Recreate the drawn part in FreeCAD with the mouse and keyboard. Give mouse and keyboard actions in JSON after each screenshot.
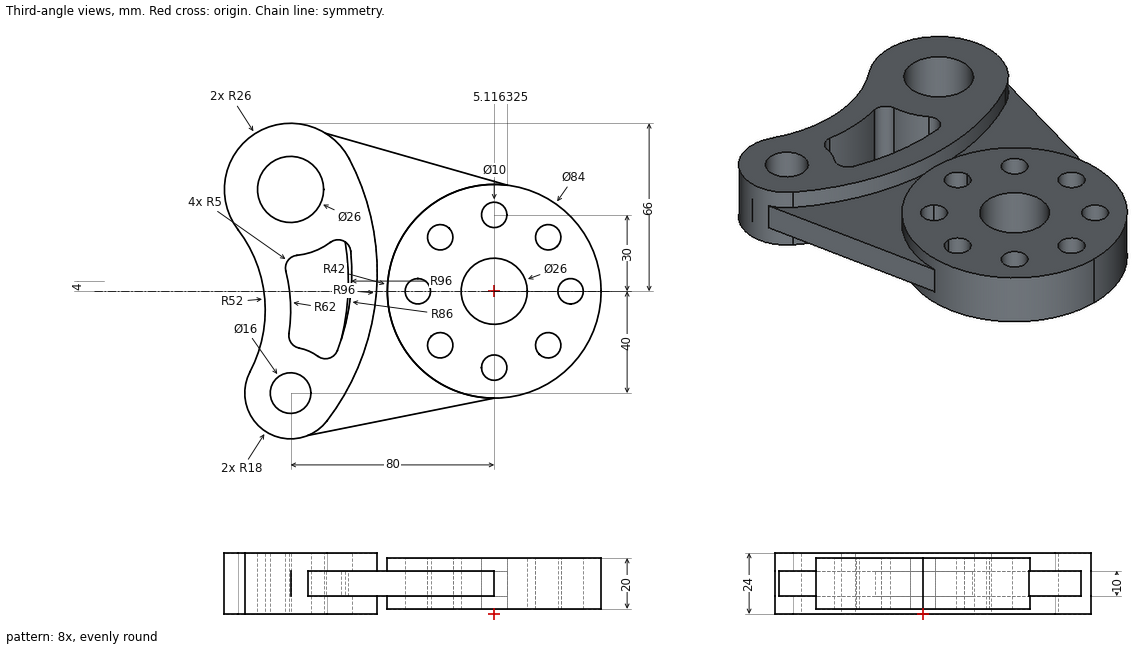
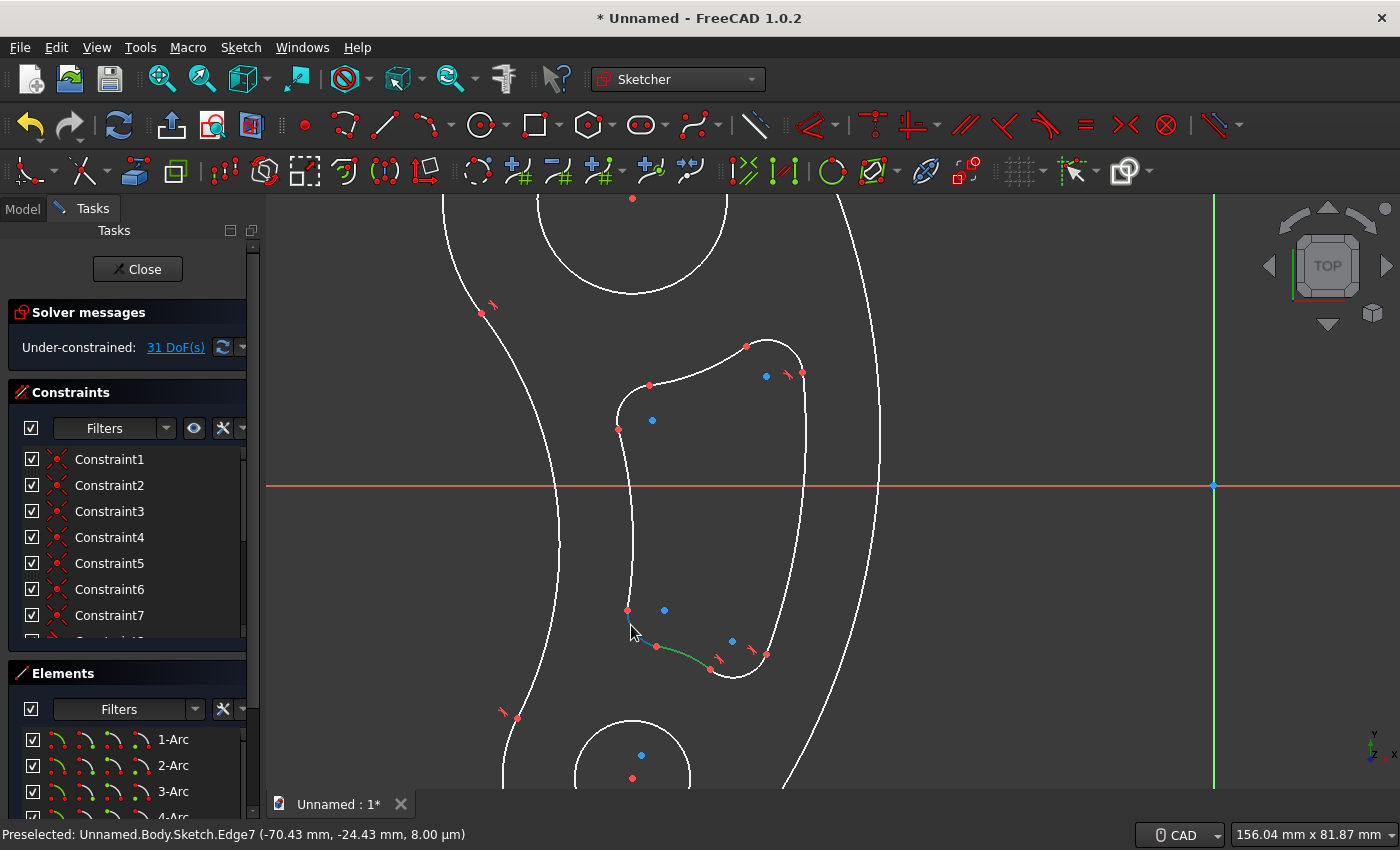
{"action": "left_click", "coordinate": [630, 625]}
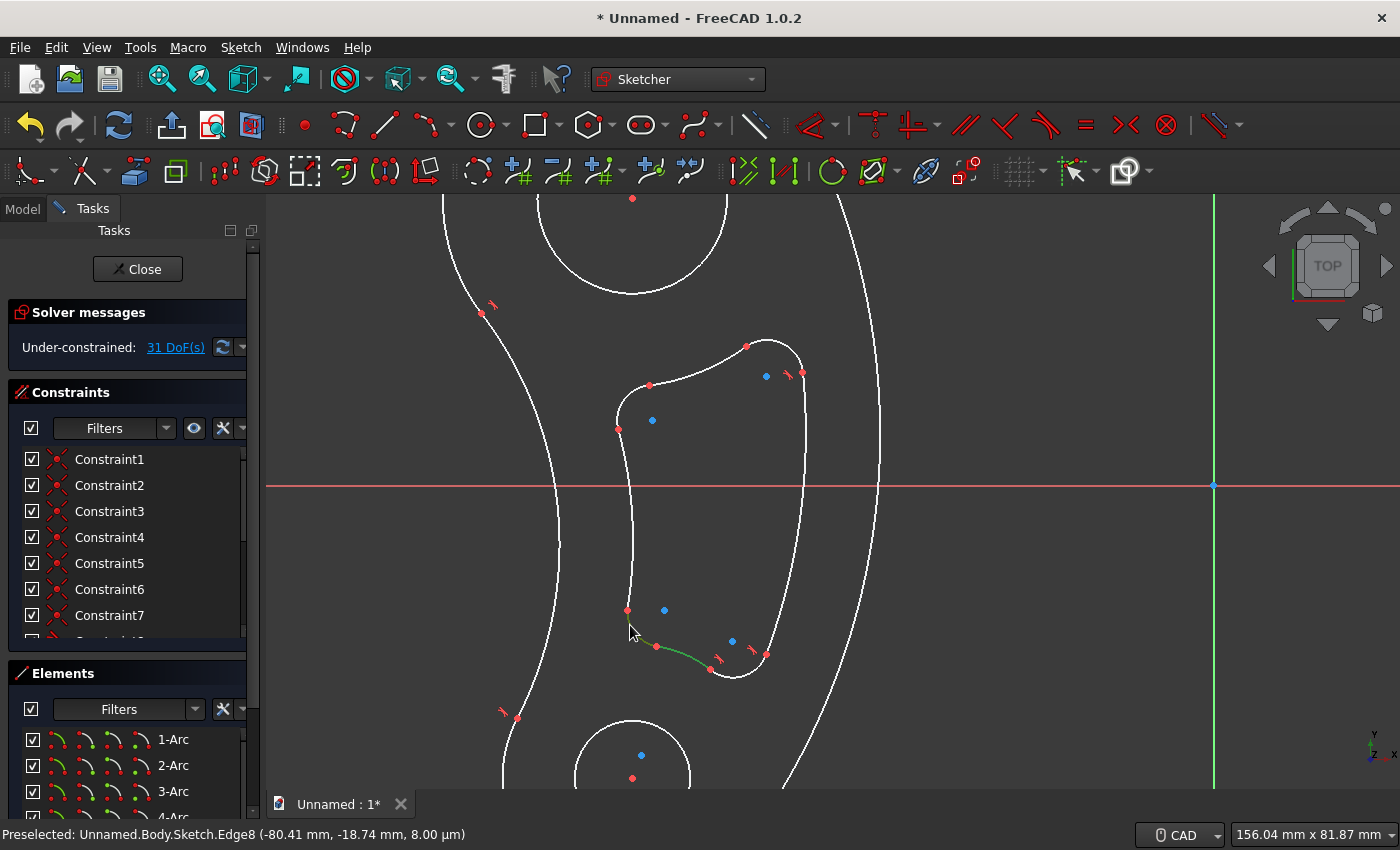
{"action": "left_click", "coordinate": [1046, 126]}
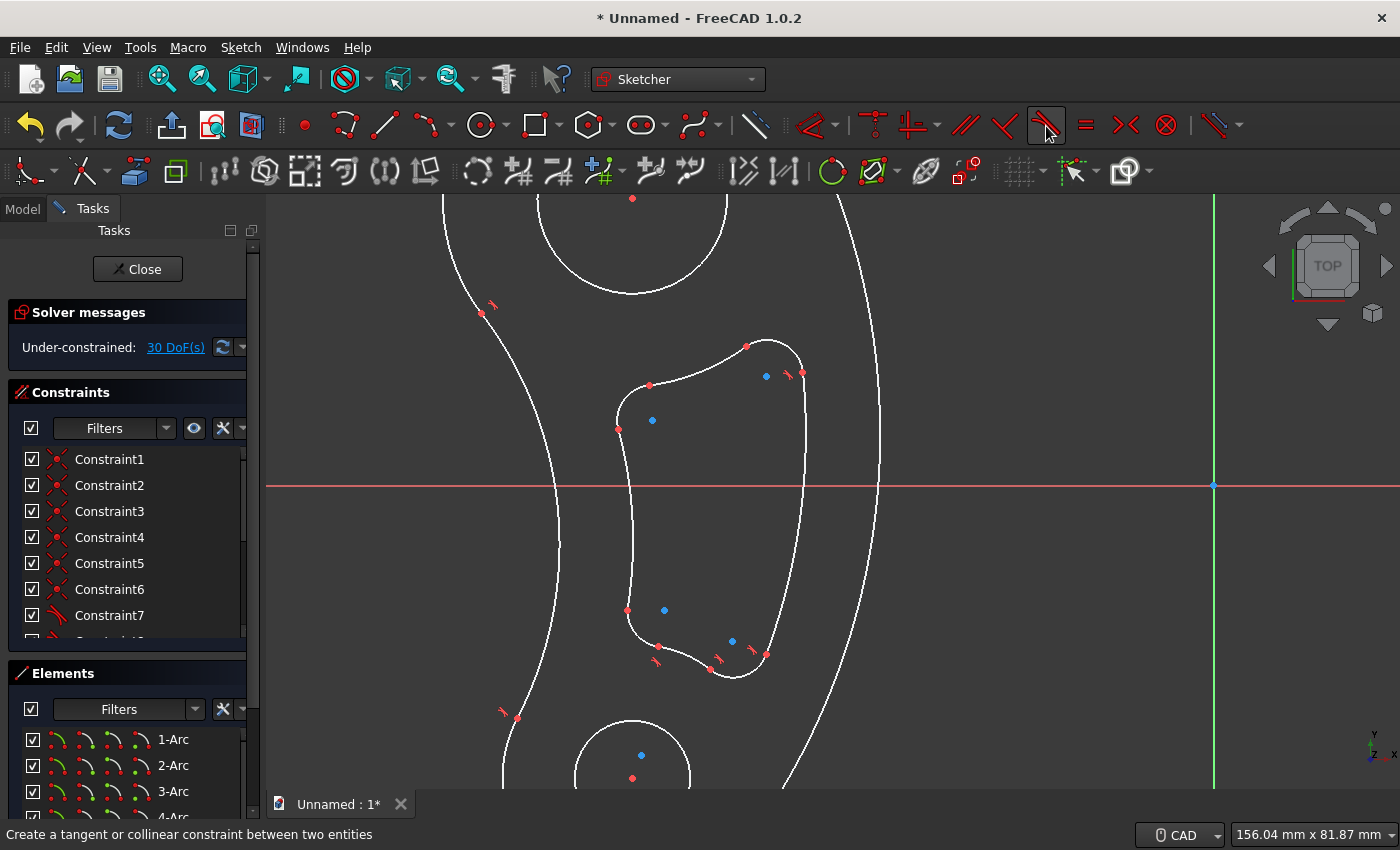
{"action": "left_click", "coordinate": [631, 625]}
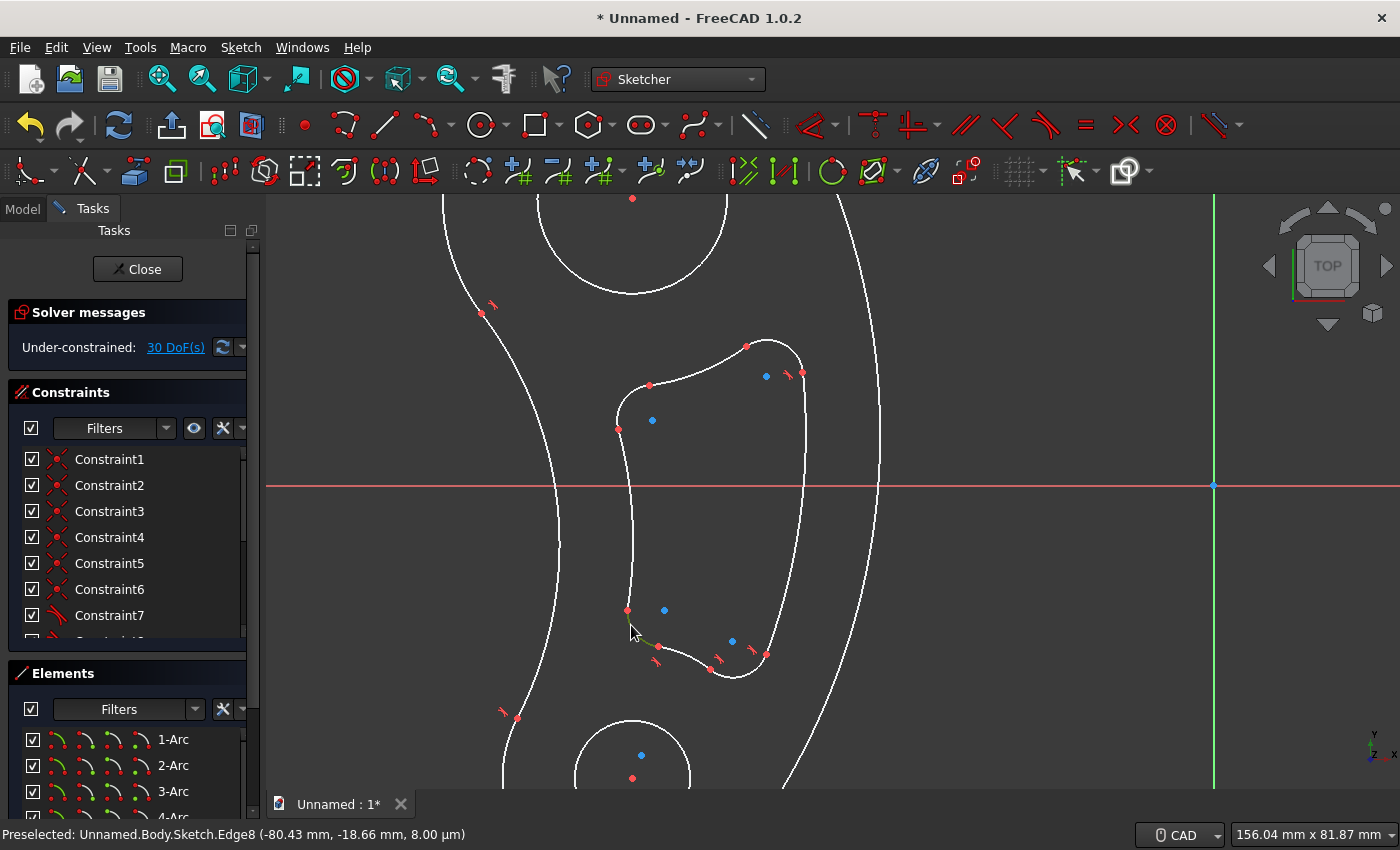
{"action": "left_click", "coordinate": [633, 556]}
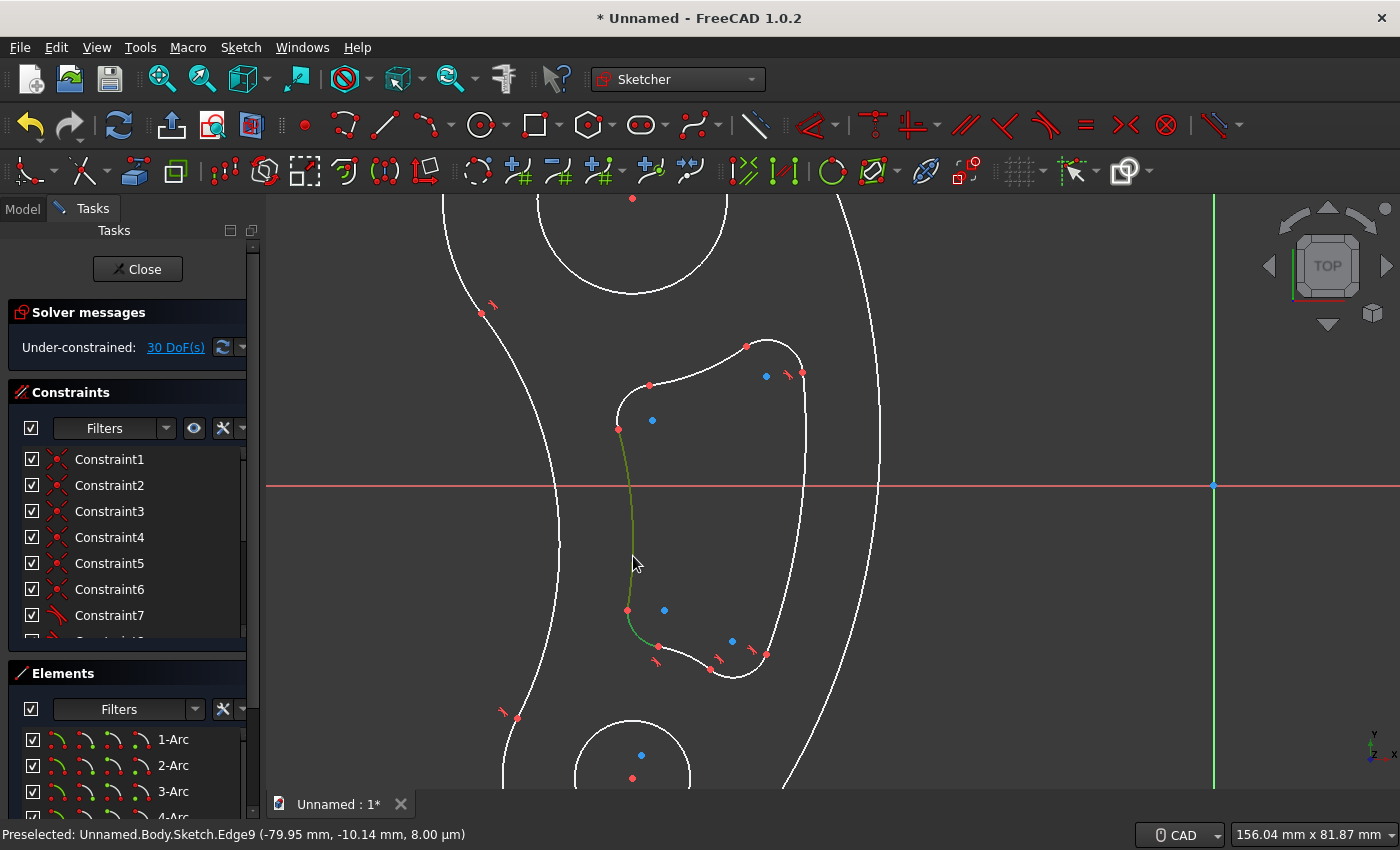
{"action": "left_click", "coordinate": [1046, 126]}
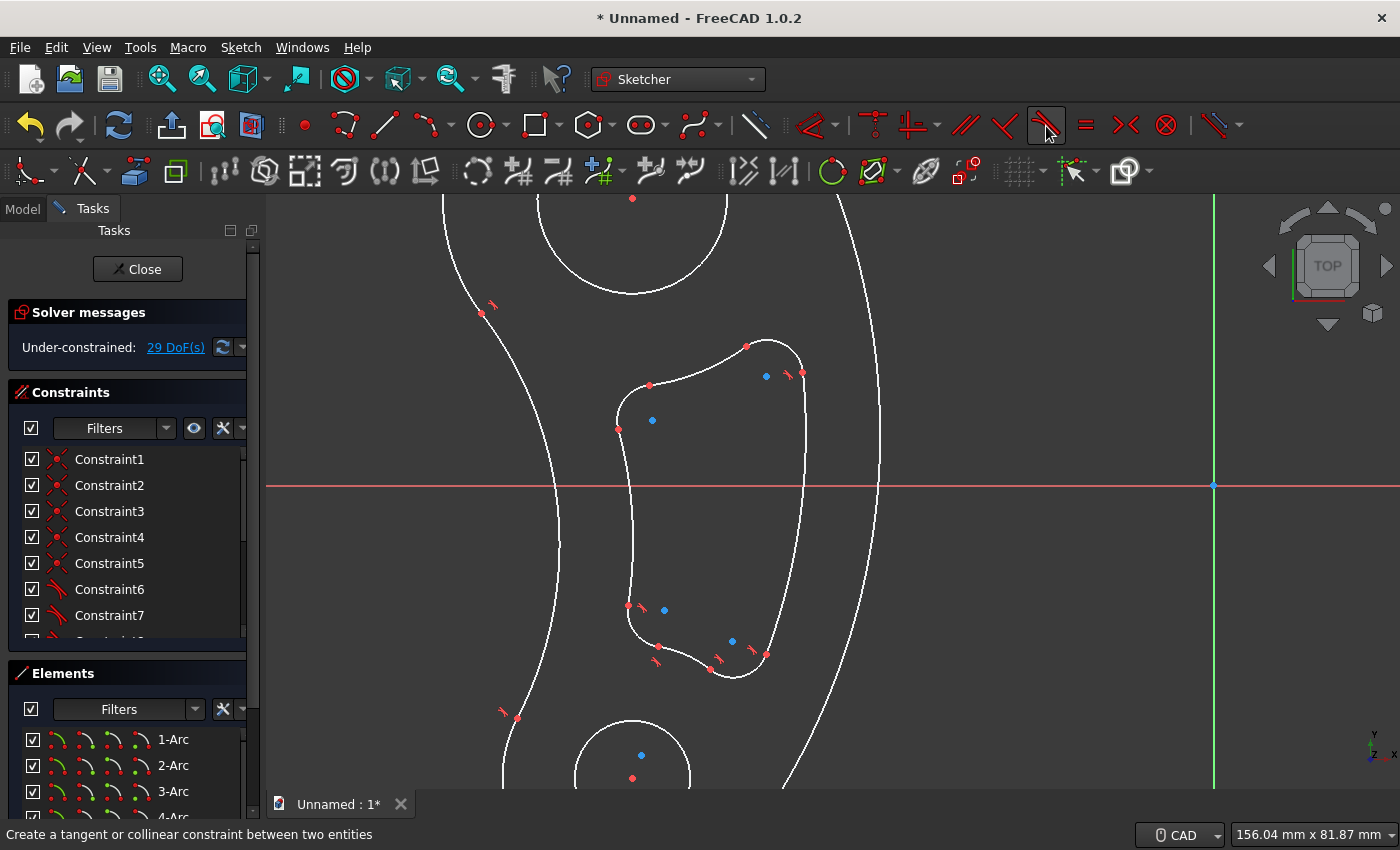
{"action": "left_click", "coordinate": [633, 552]}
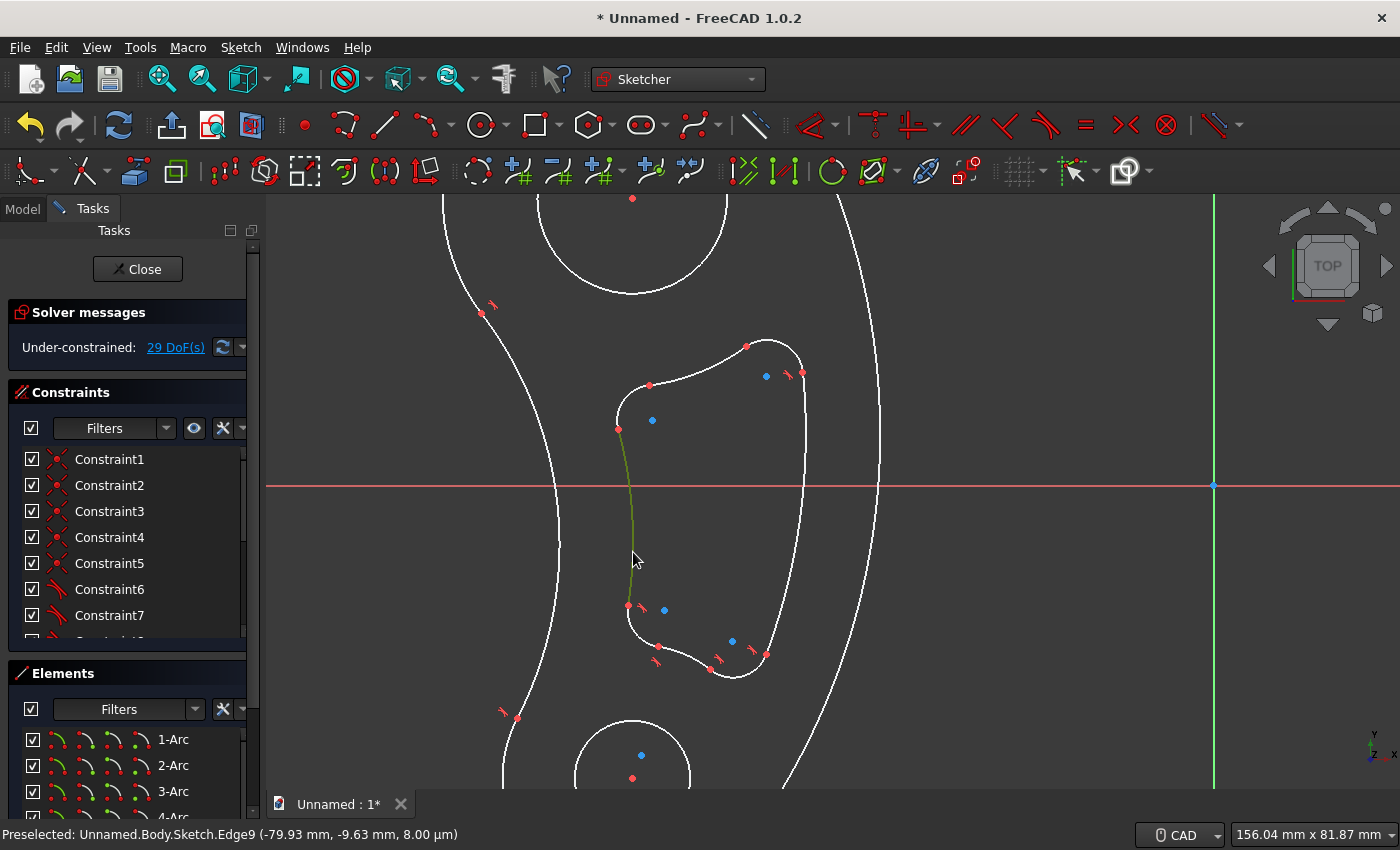
{"action": "left_click", "coordinate": [632, 392]}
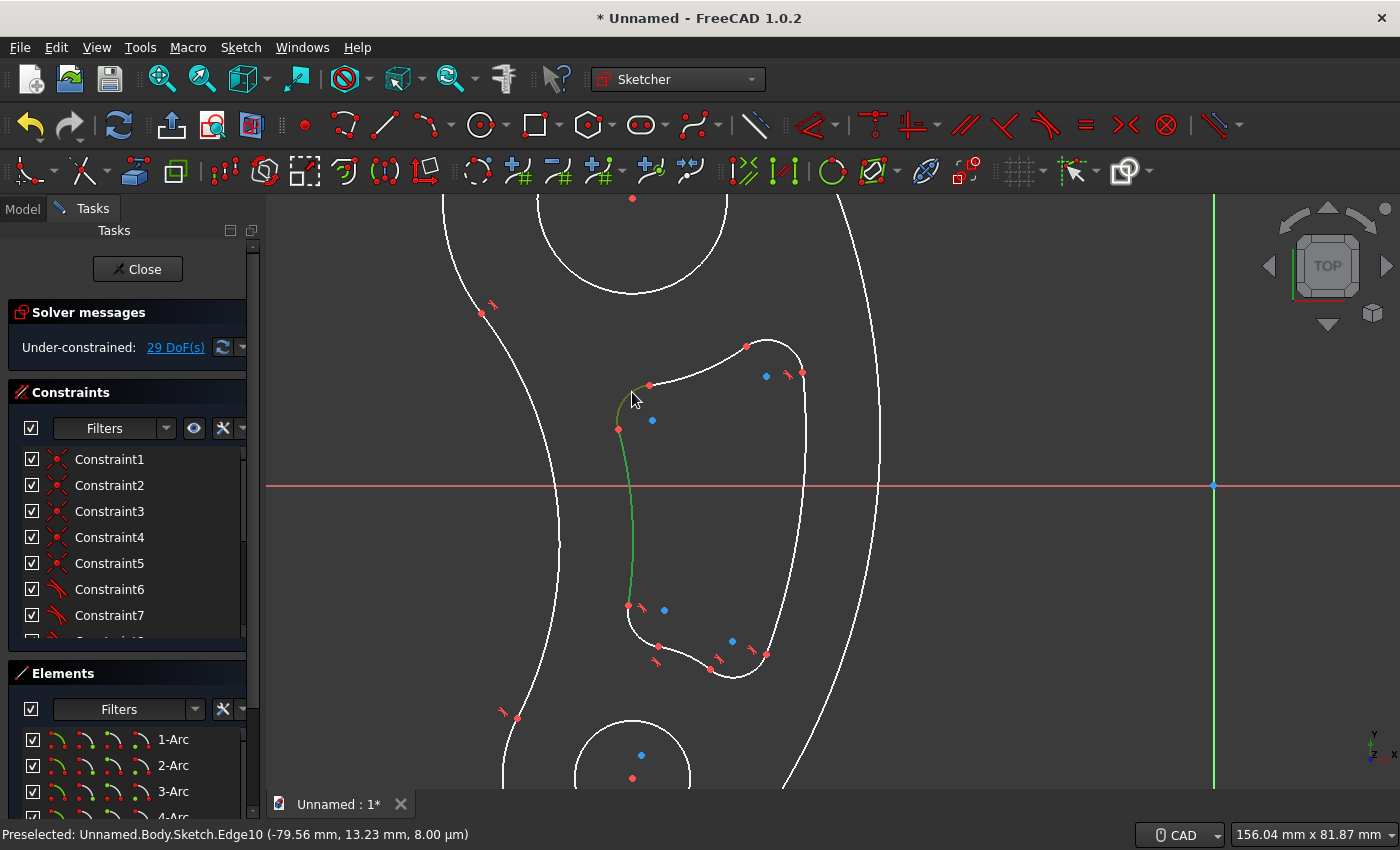
{"action": "left_click", "coordinate": [1046, 126]}